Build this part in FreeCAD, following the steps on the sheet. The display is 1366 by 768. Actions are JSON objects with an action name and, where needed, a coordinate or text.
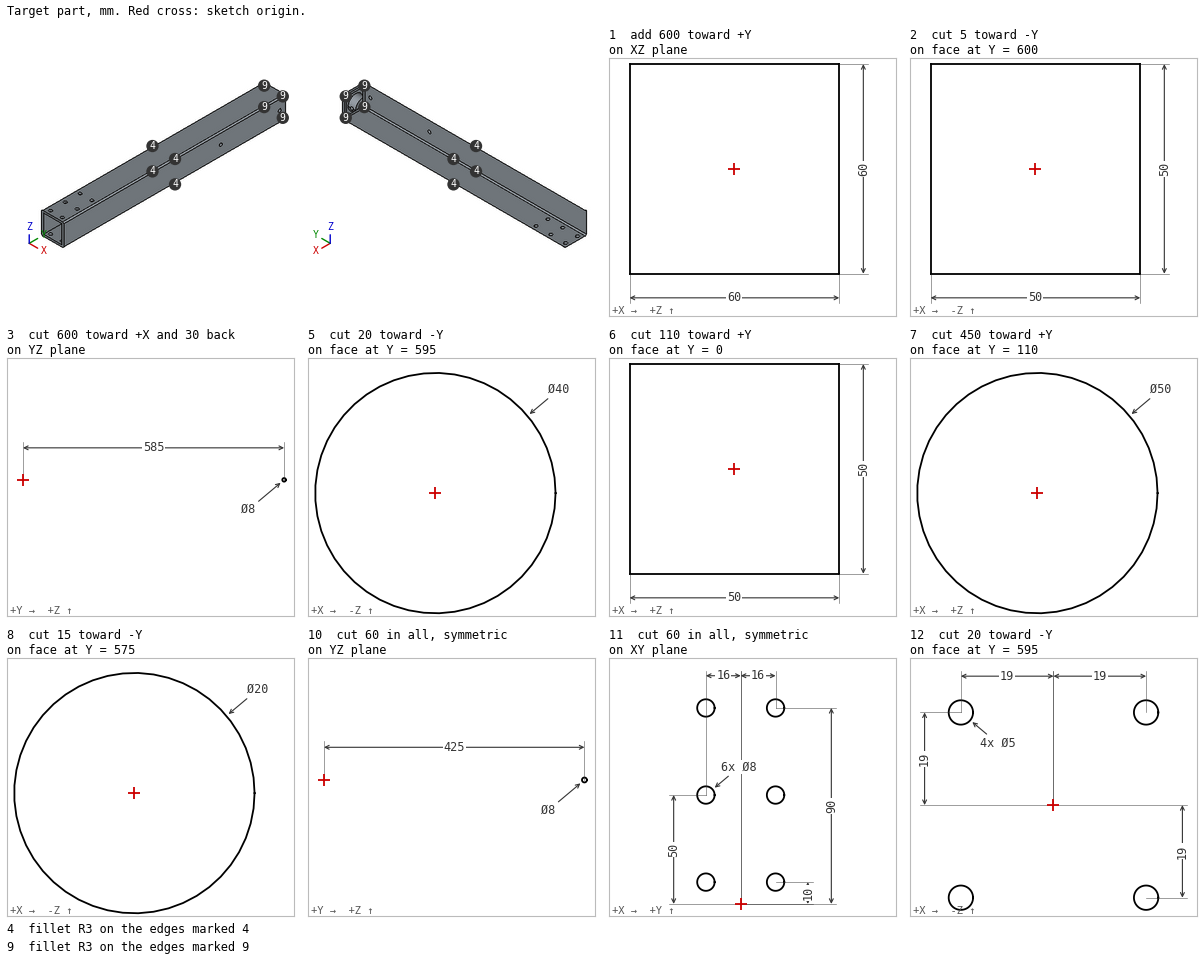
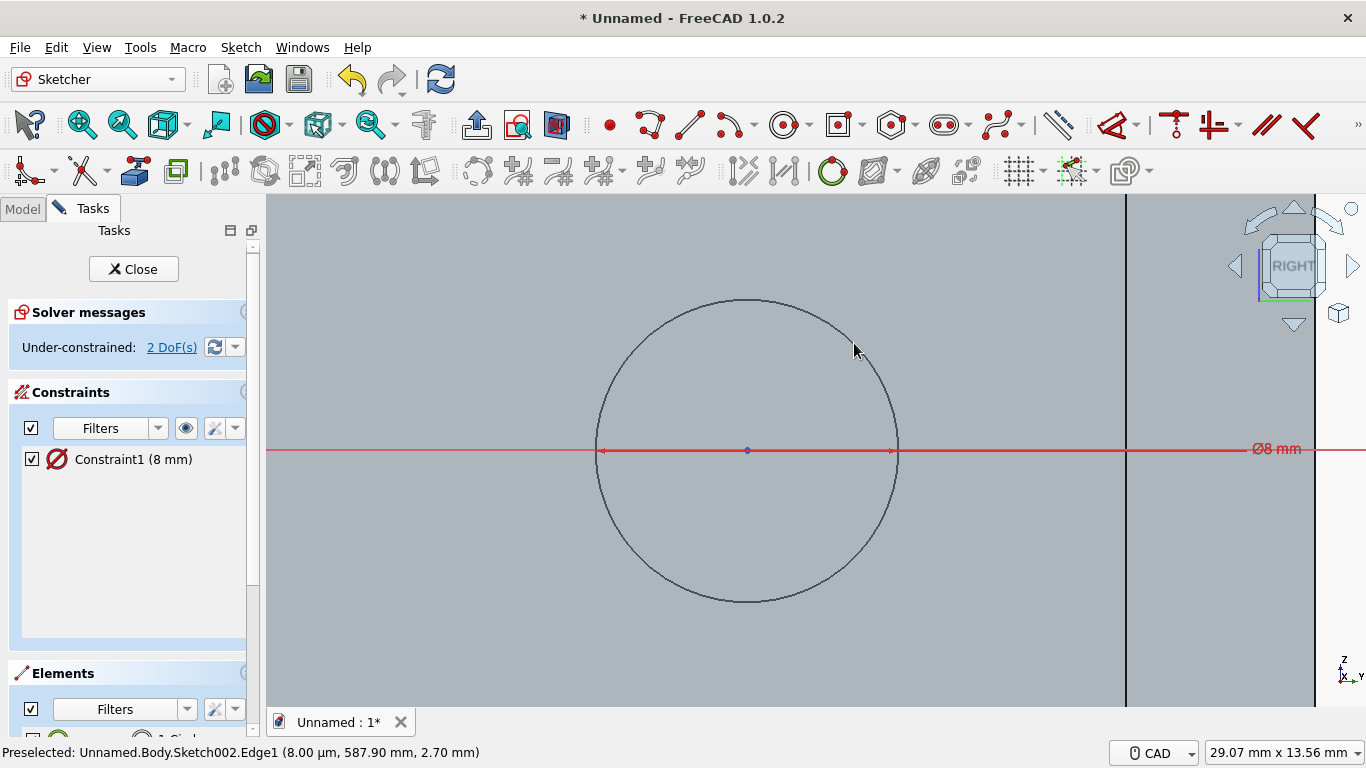
{"action": "left_click", "coordinate": [747, 451]}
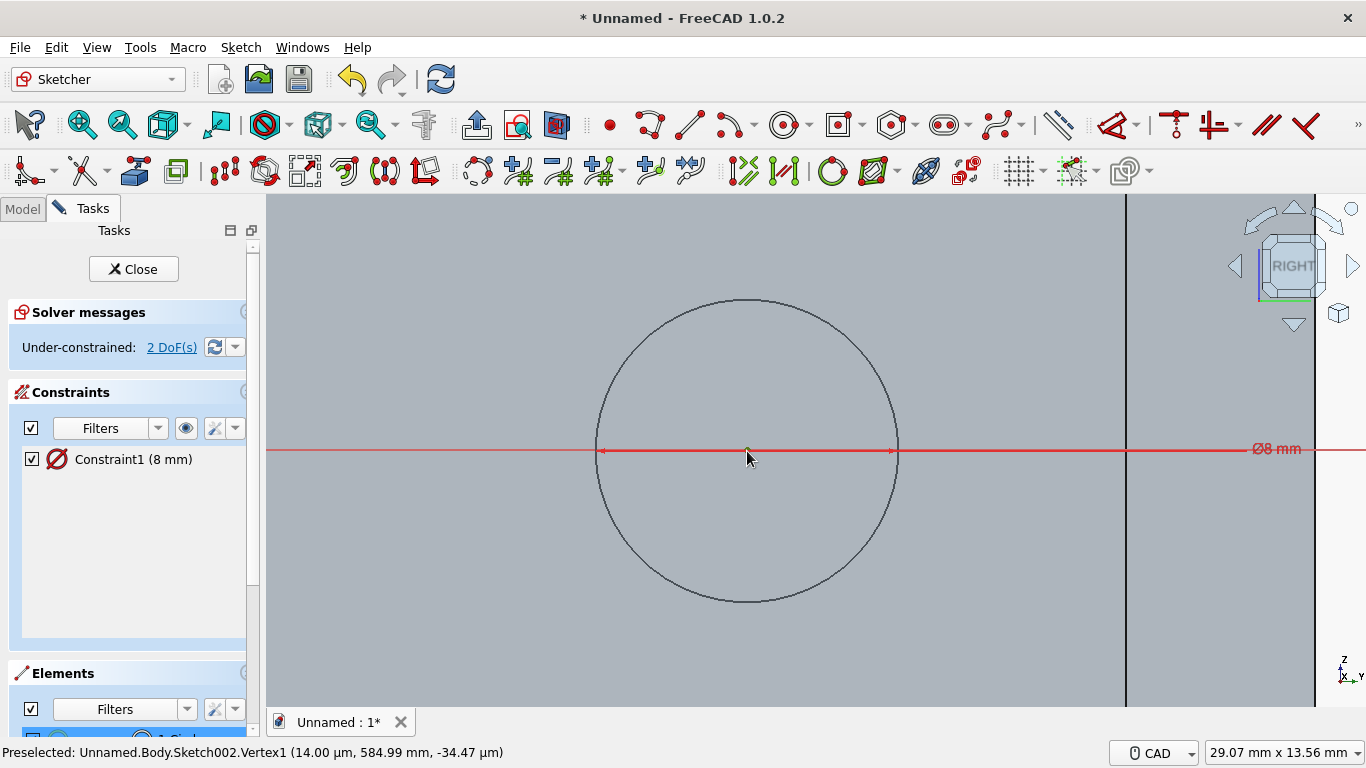
{"action": "left_click", "coordinate": [359, 450]}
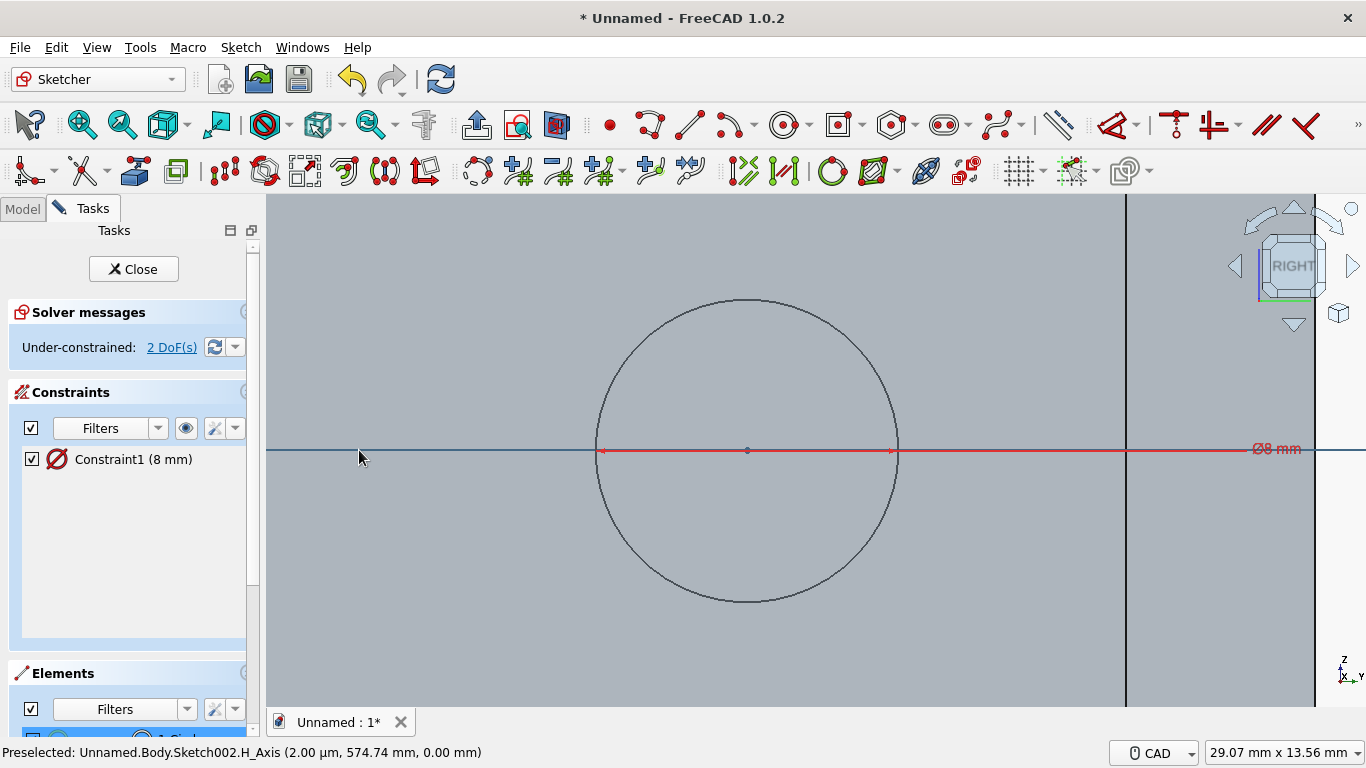
{"action": "left_click", "coordinate": [1174, 126]}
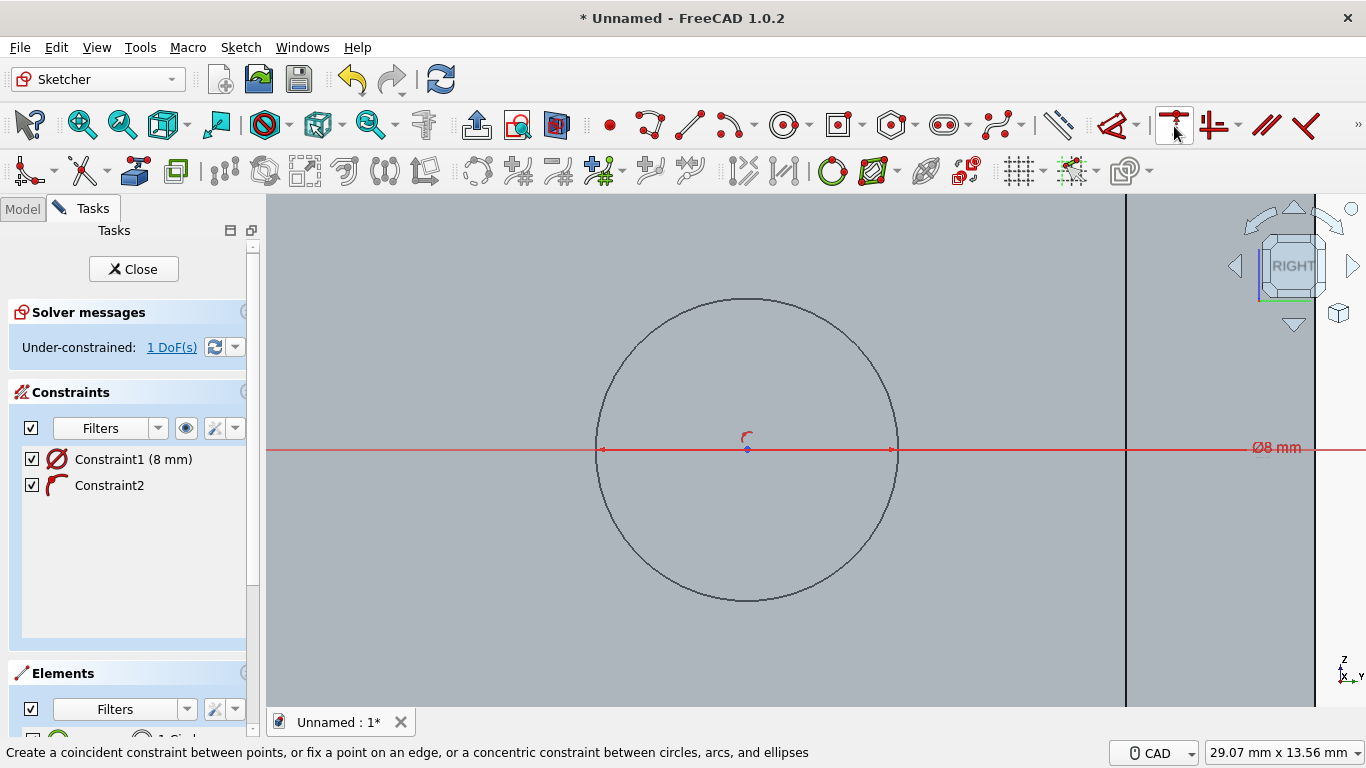
{"action": "left_click", "coordinate": [747, 450]}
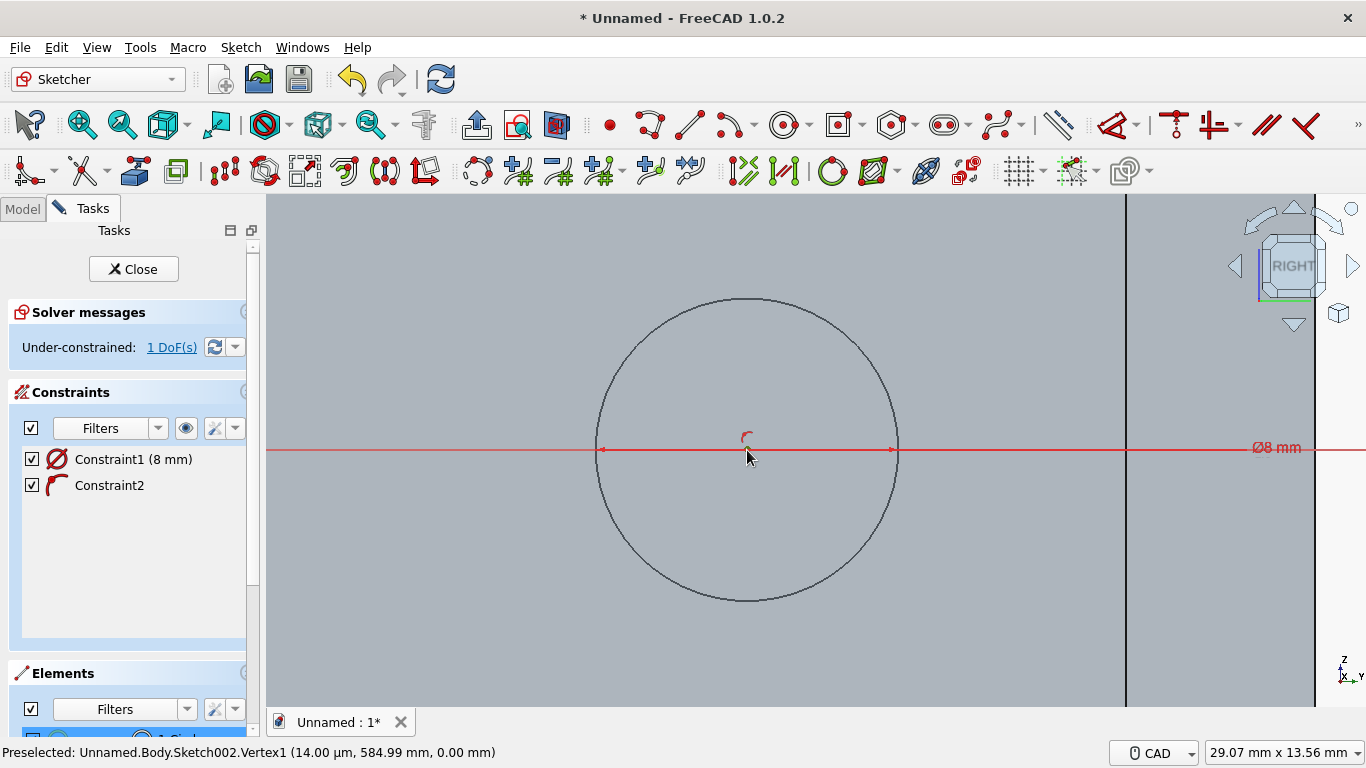
{"action": "left_click", "coordinate": [1138, 126]}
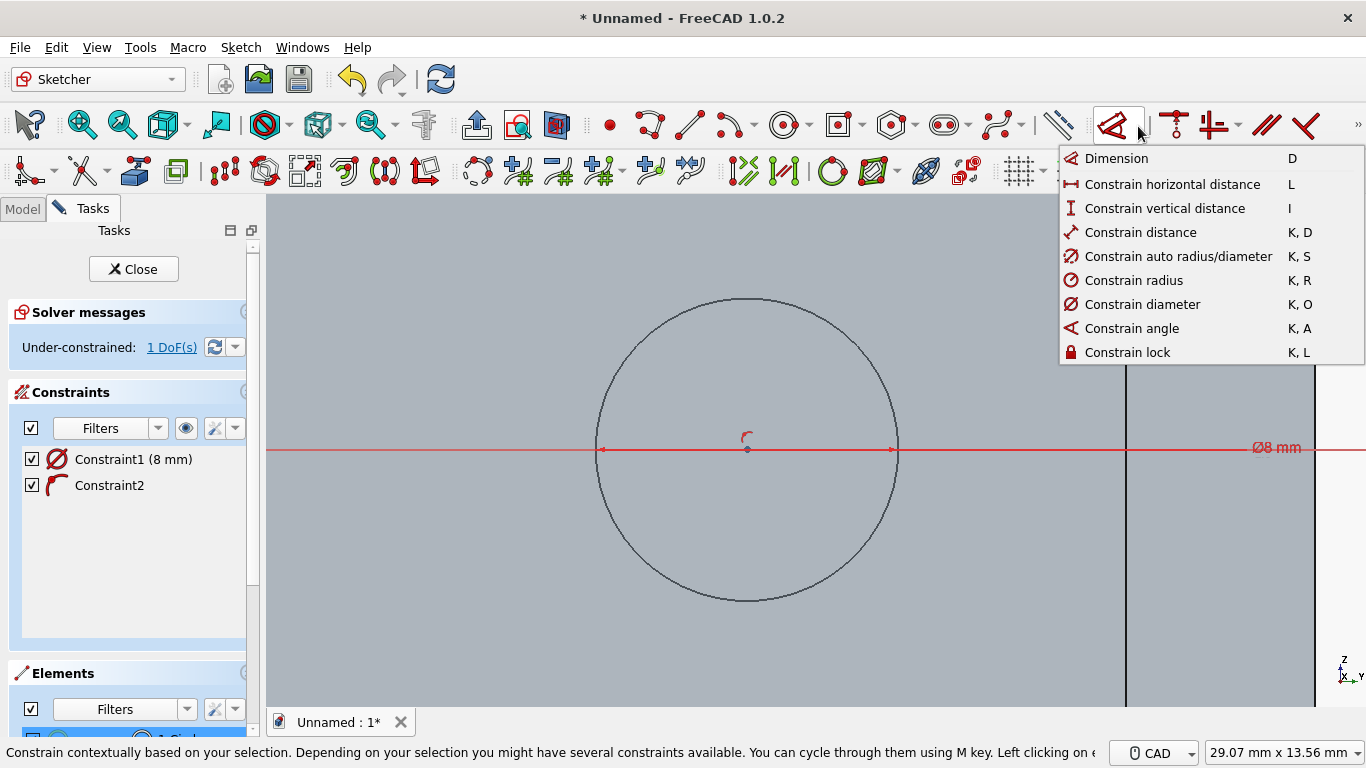
{"action": "left_click", "coordinate": [1212, 184]}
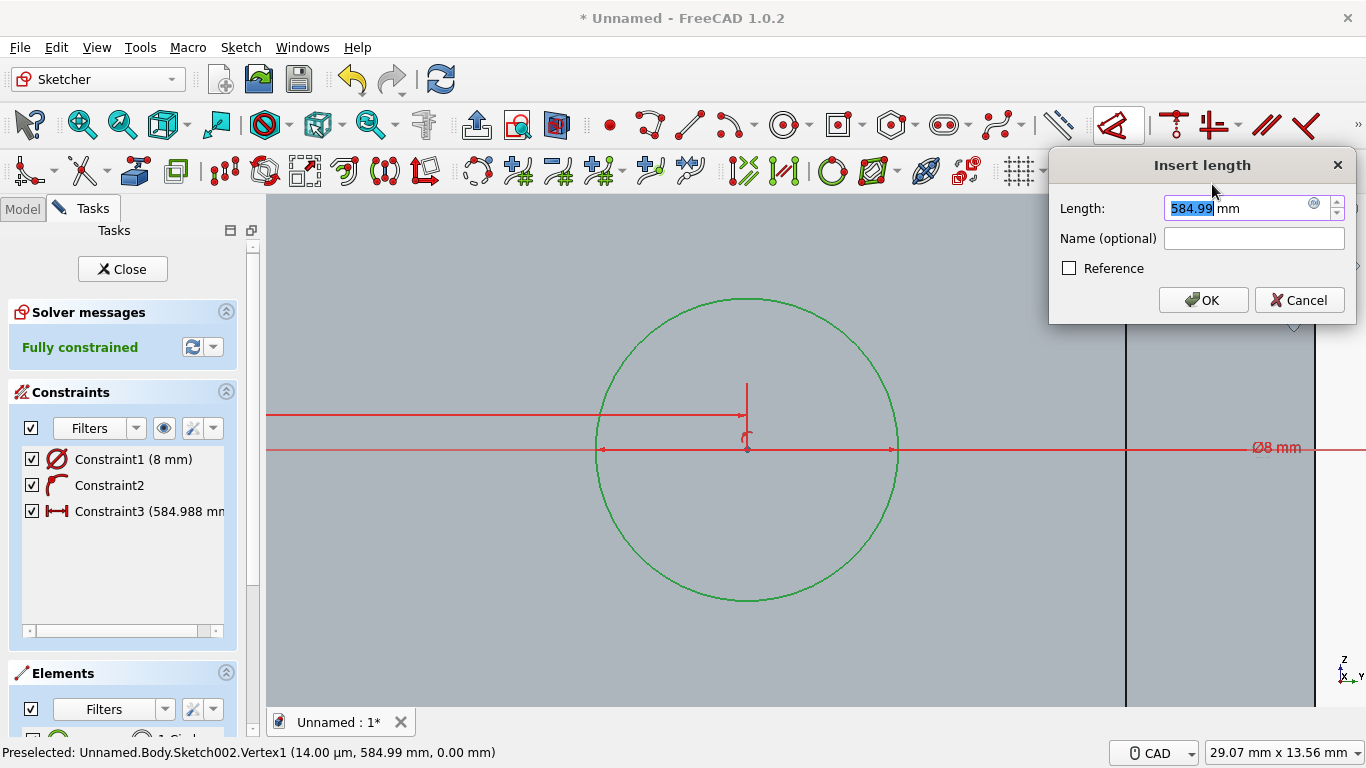
{"action": "type", "text": "585"}
{"action": "key", "text": "Return"}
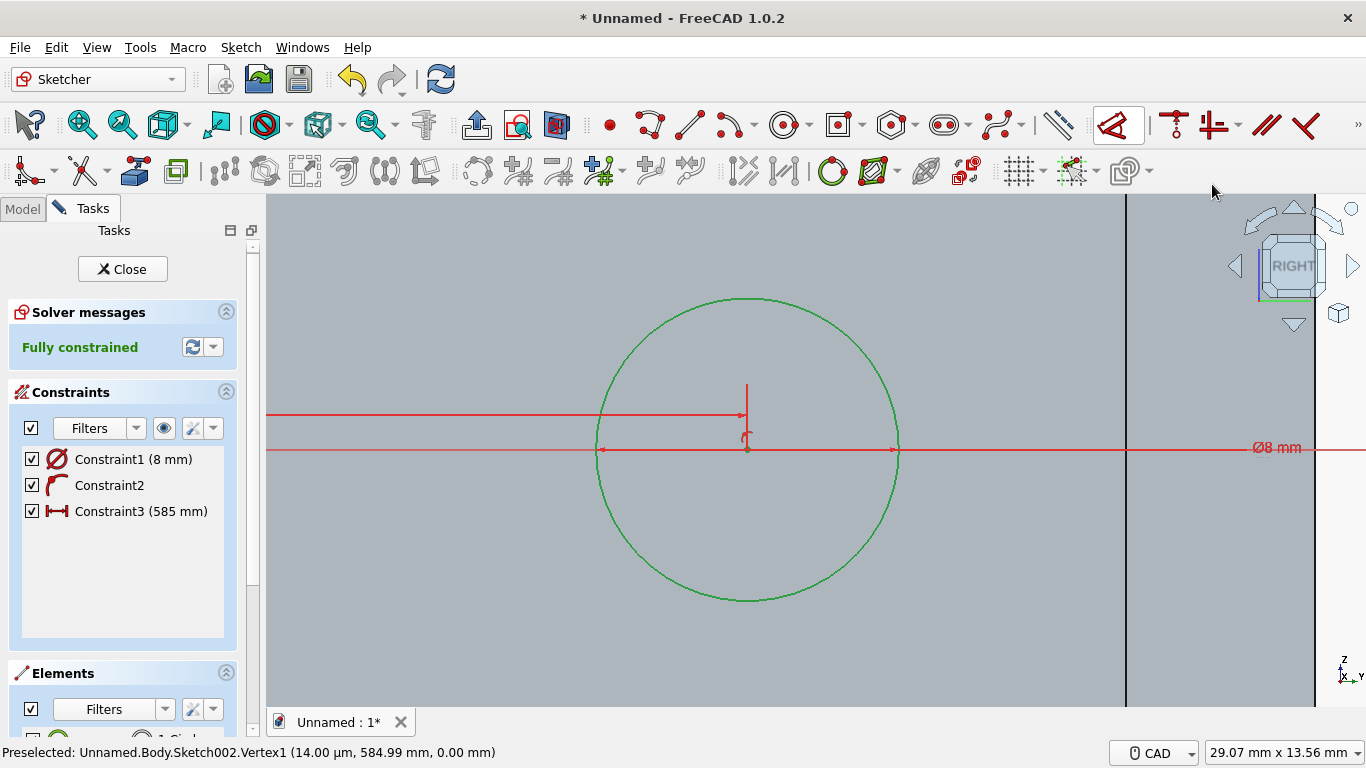
{"action": "left_click", "coordinate": [123, 269]}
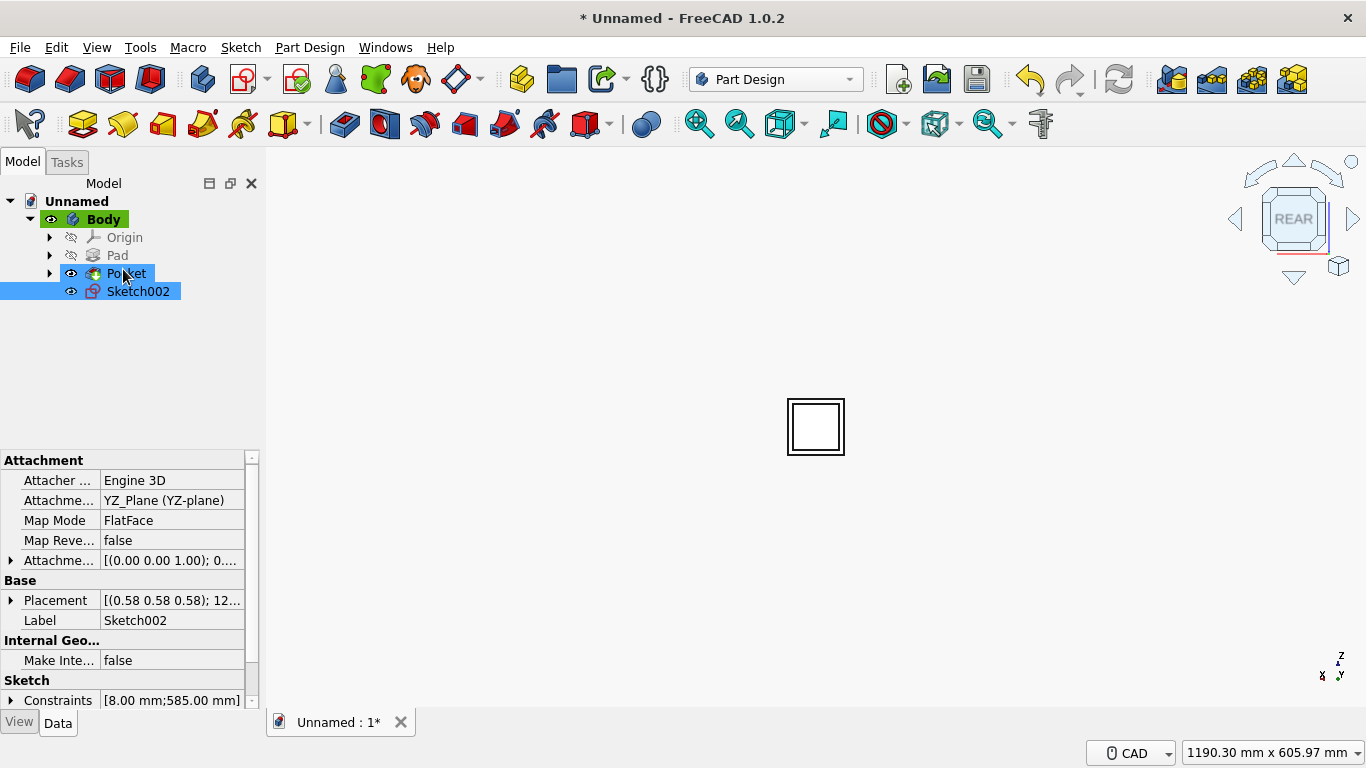
{"action": "left_click", "coordinate": [346, 124]}